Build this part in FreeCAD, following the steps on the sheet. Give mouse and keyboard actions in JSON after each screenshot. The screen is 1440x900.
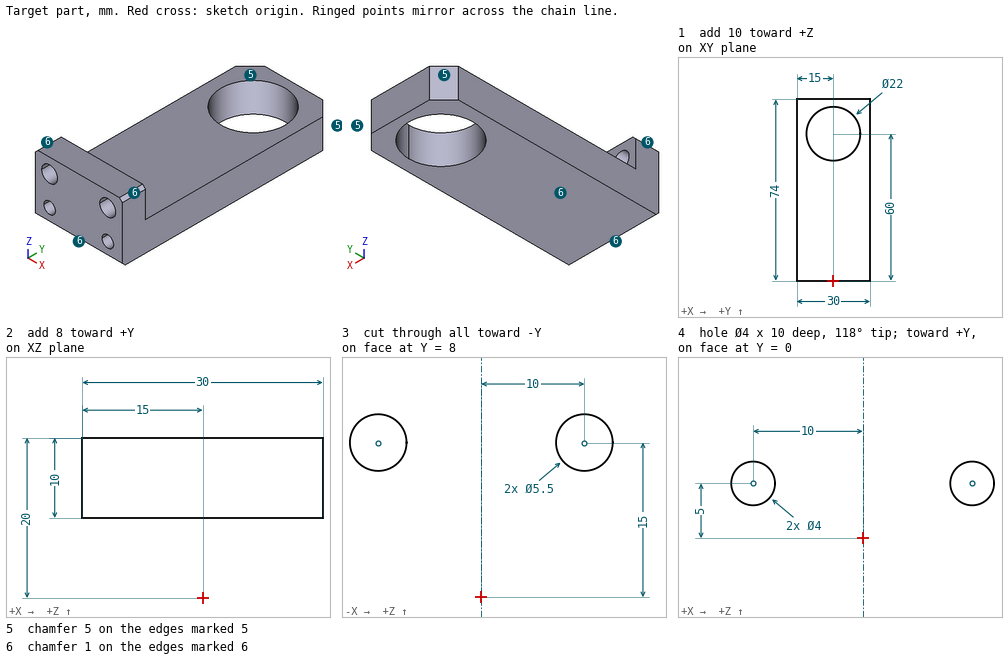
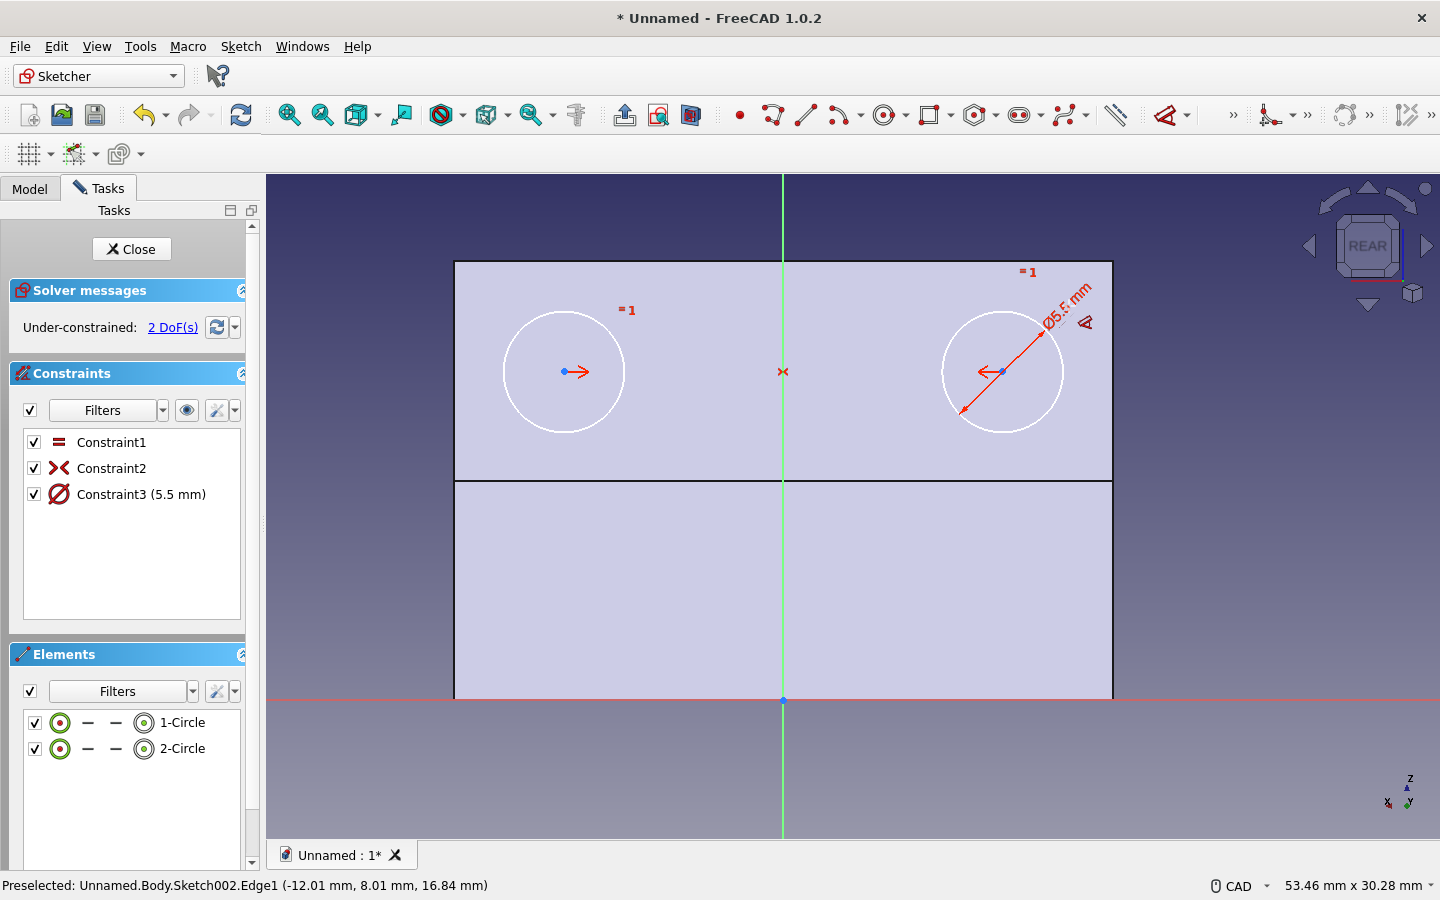
{"action": "left_click", "coordinate": [1003, 372]}
{"action": "left_click", "coordinate": [893, 734]}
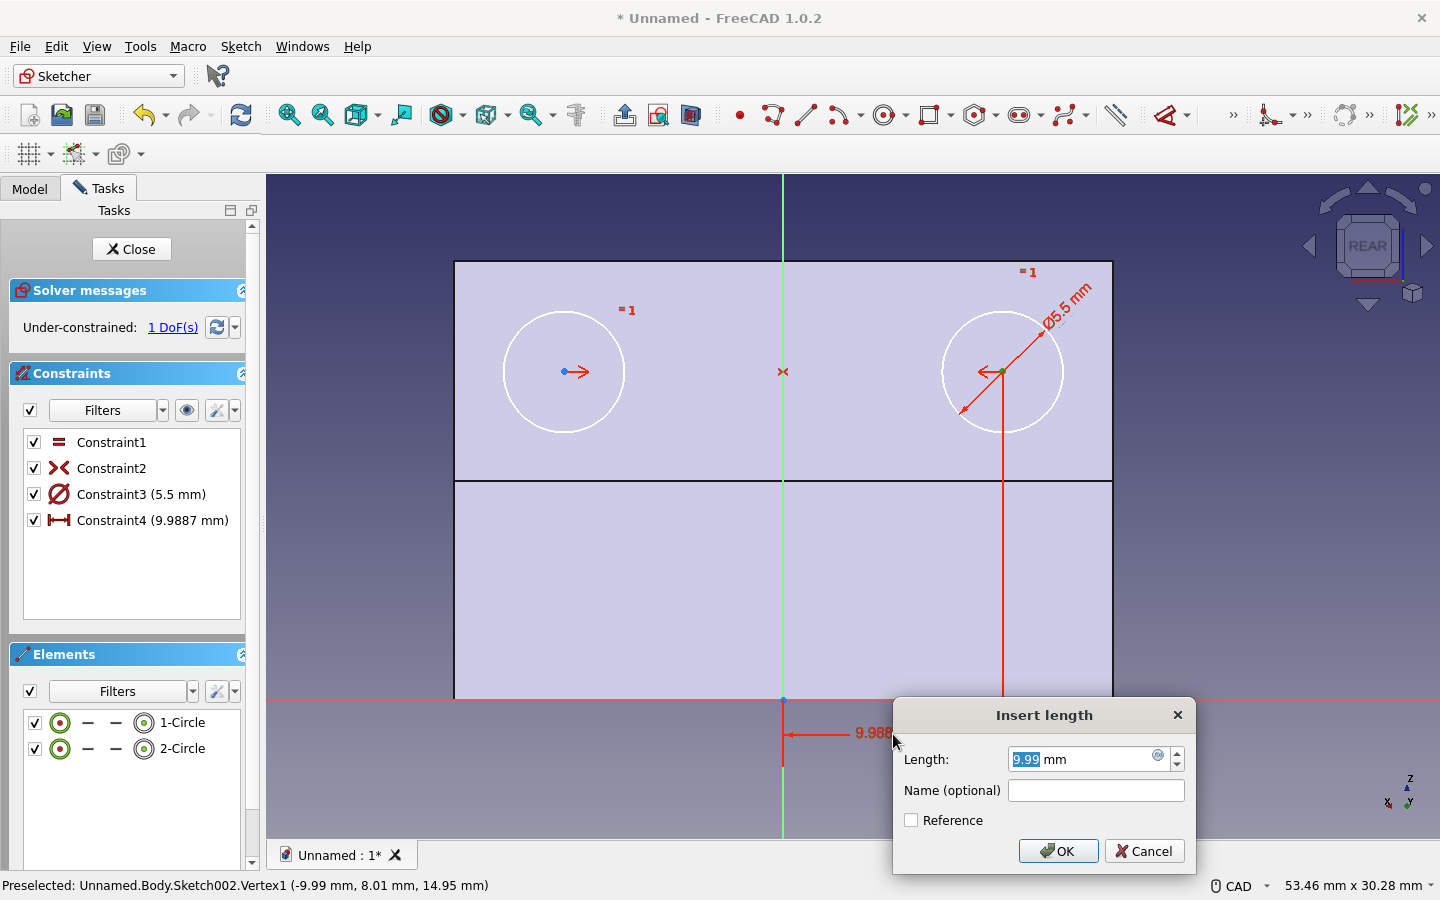
{"action": "type", "text": "10"}
{"action": "key", "text": "Return"}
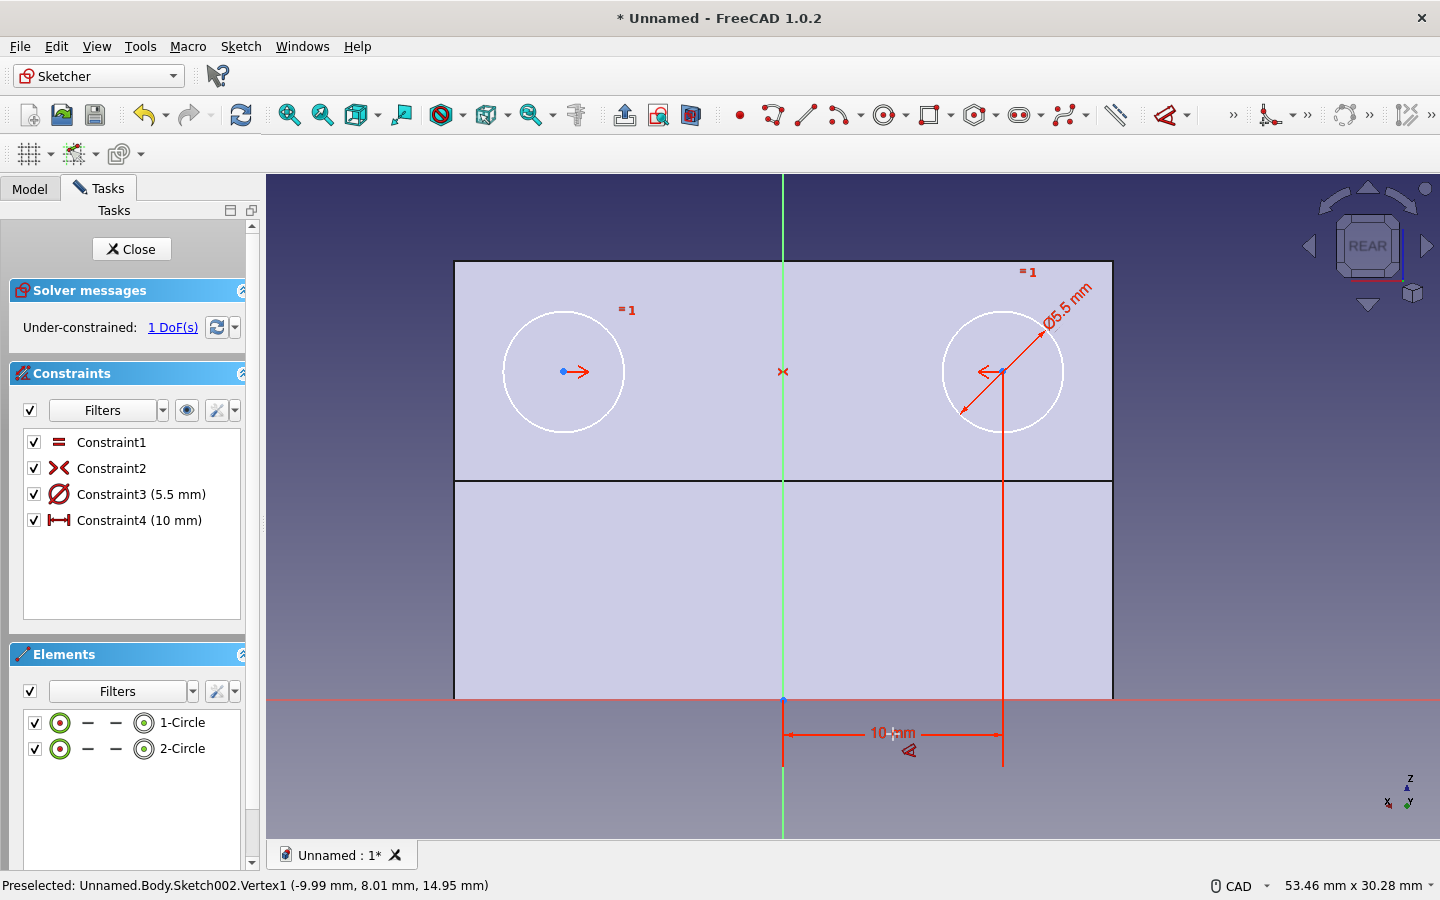
{"action": "left_click", "coordinate": [1003, 372]}
{"action": "left_click", "coordinate": [1037, 536]}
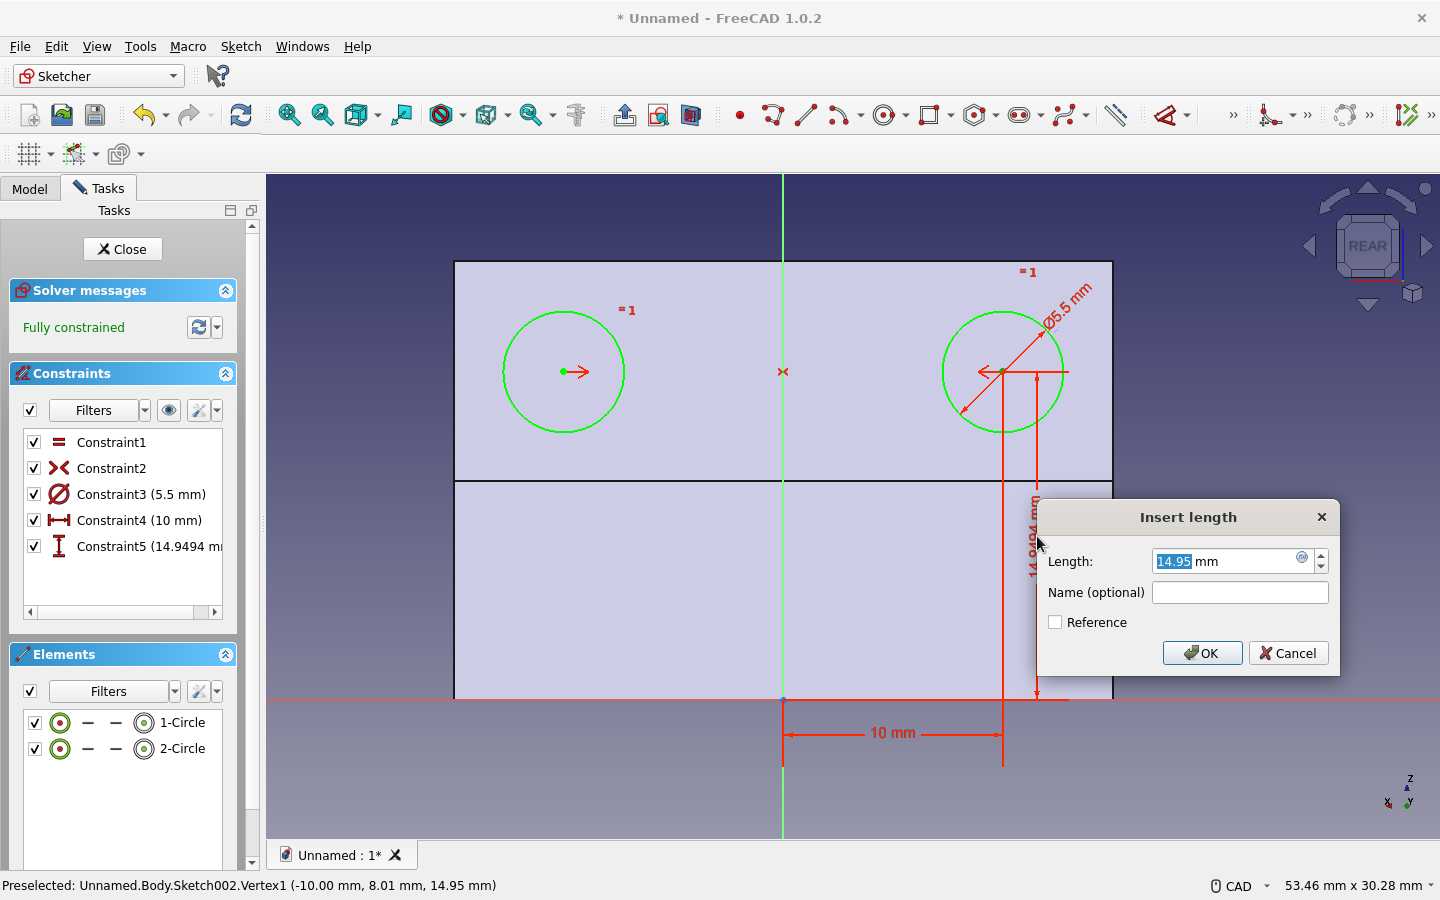
{"action": "type", "text": "15"}
{"action": "key", "text": "Return"}
{"action": "key", "text": "Escape"}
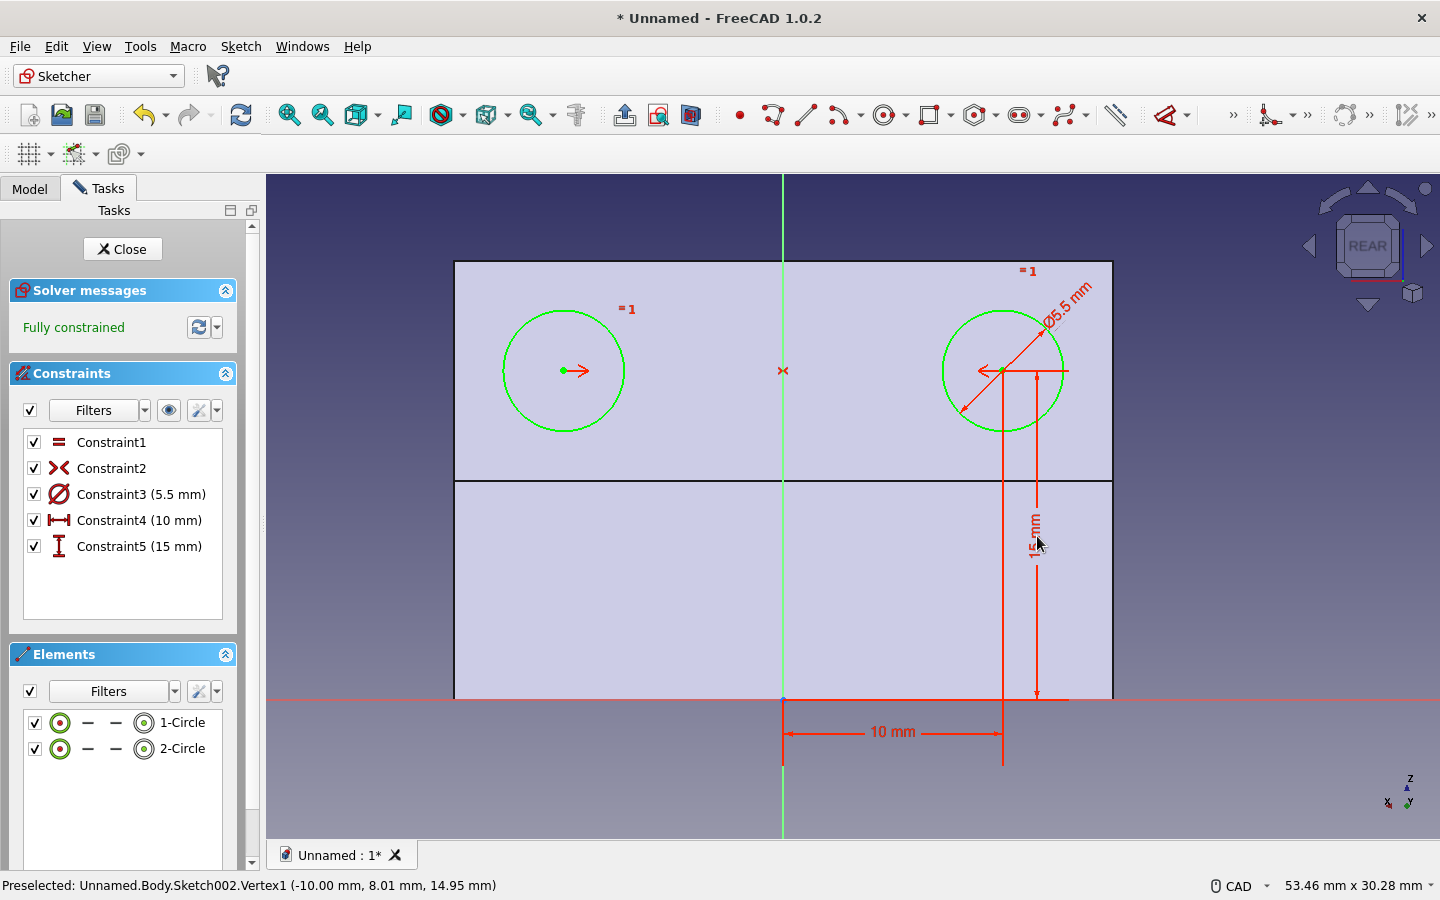
{"action": "left_click", "coordinate": [123, 249]}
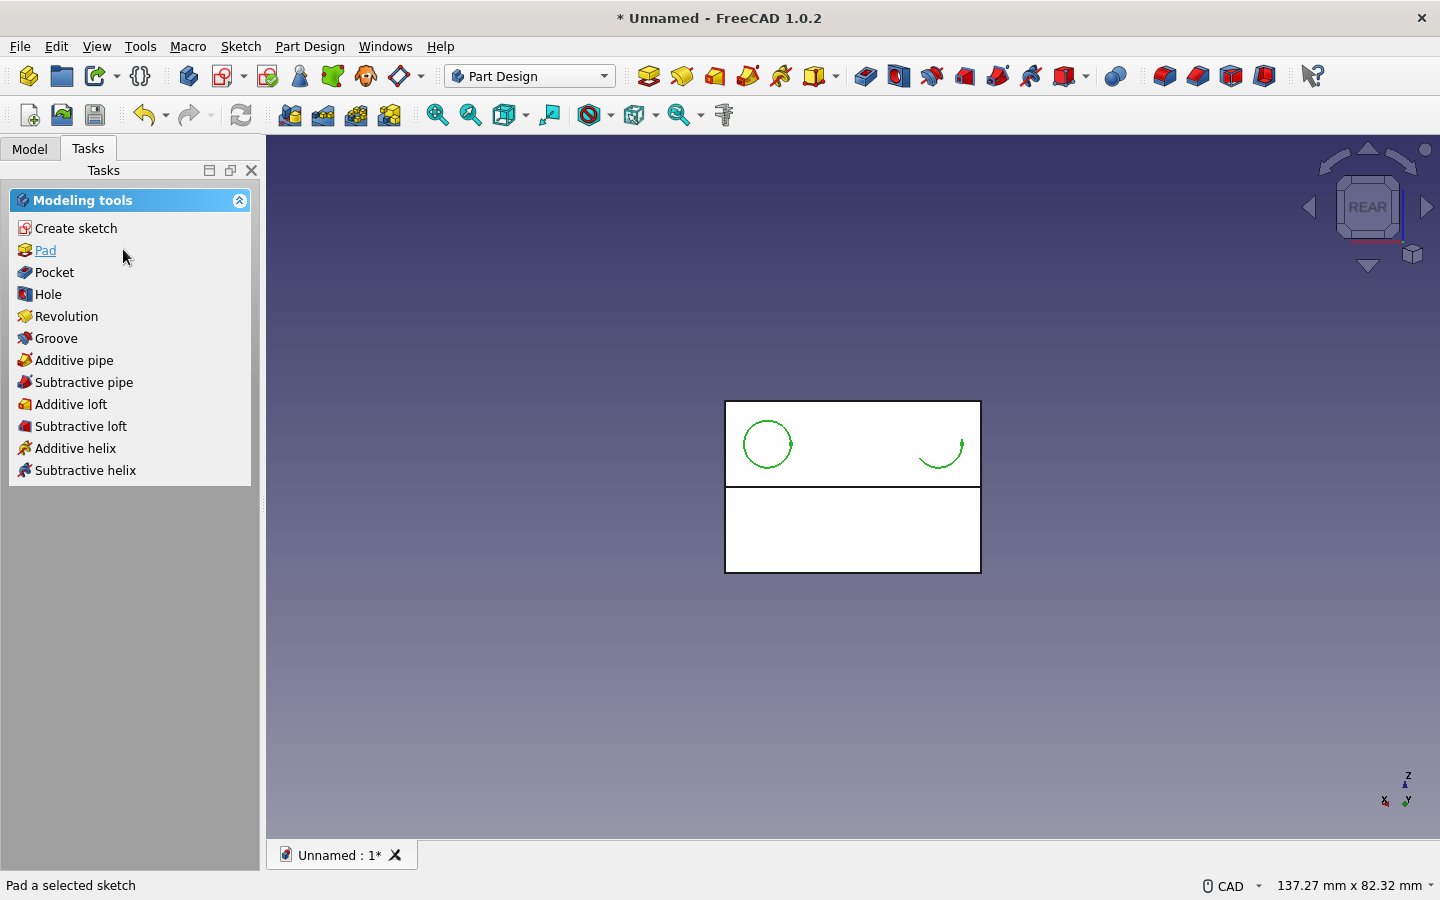
{"action": "left_click", "coordinate": [866, 76]}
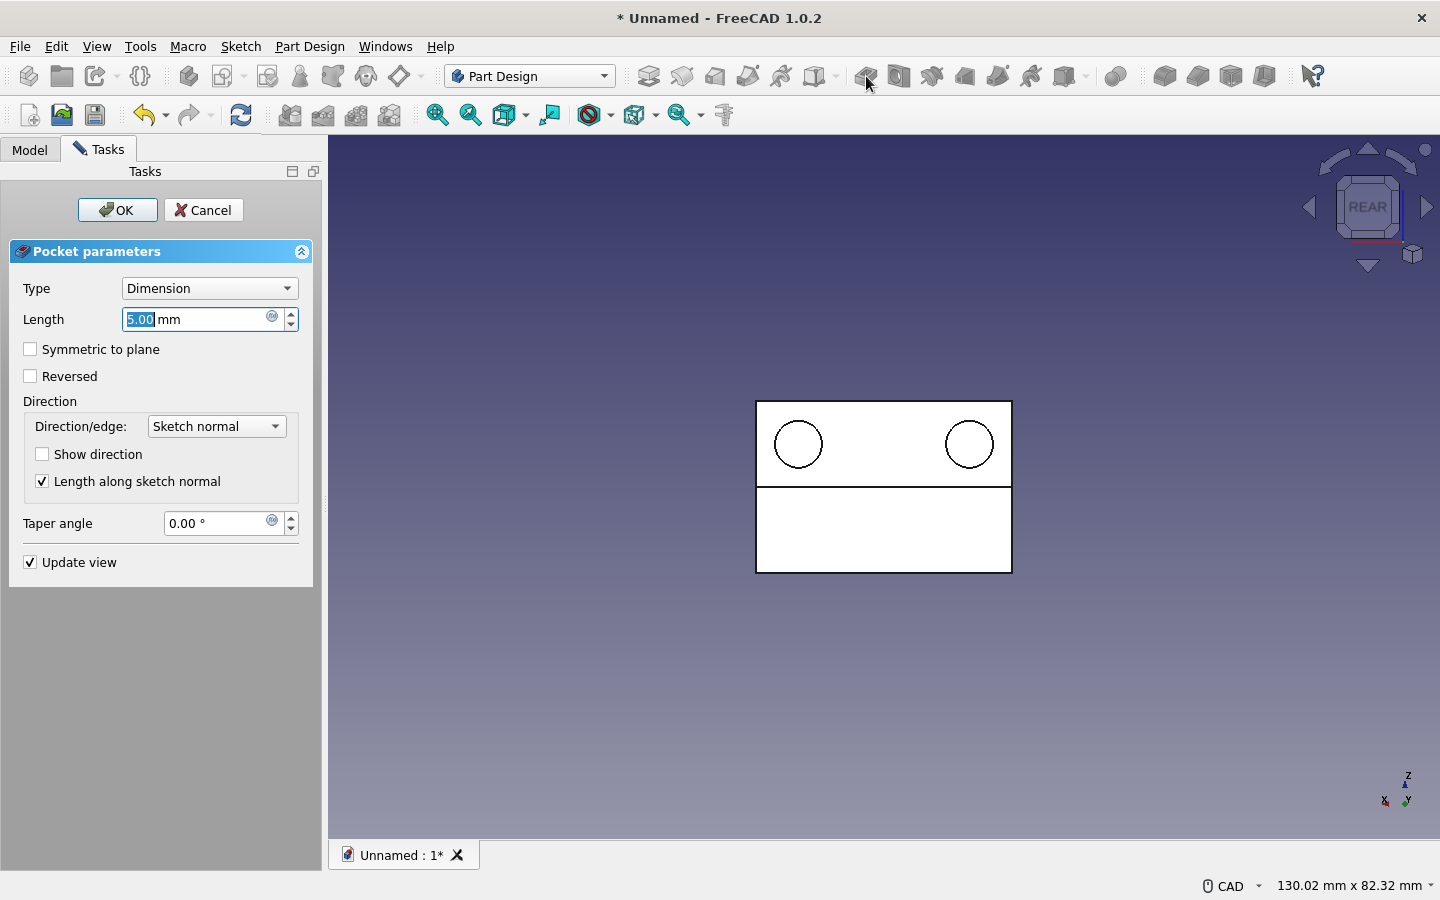
{"action": "left_click", "coordinate": [210, 288]}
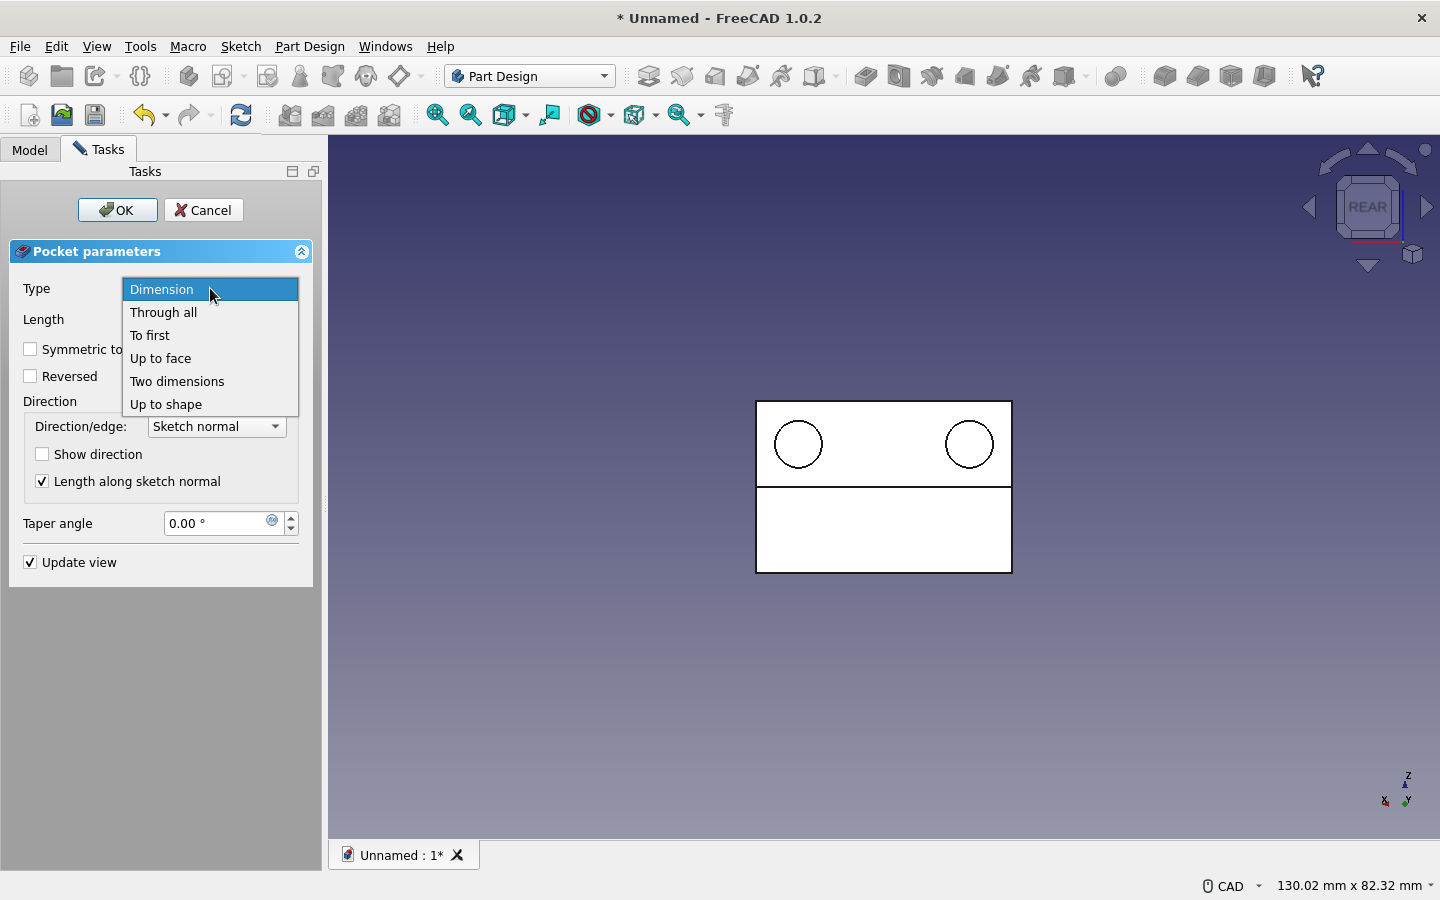
{"action": "left_click", "coordinate": [208, 312]}